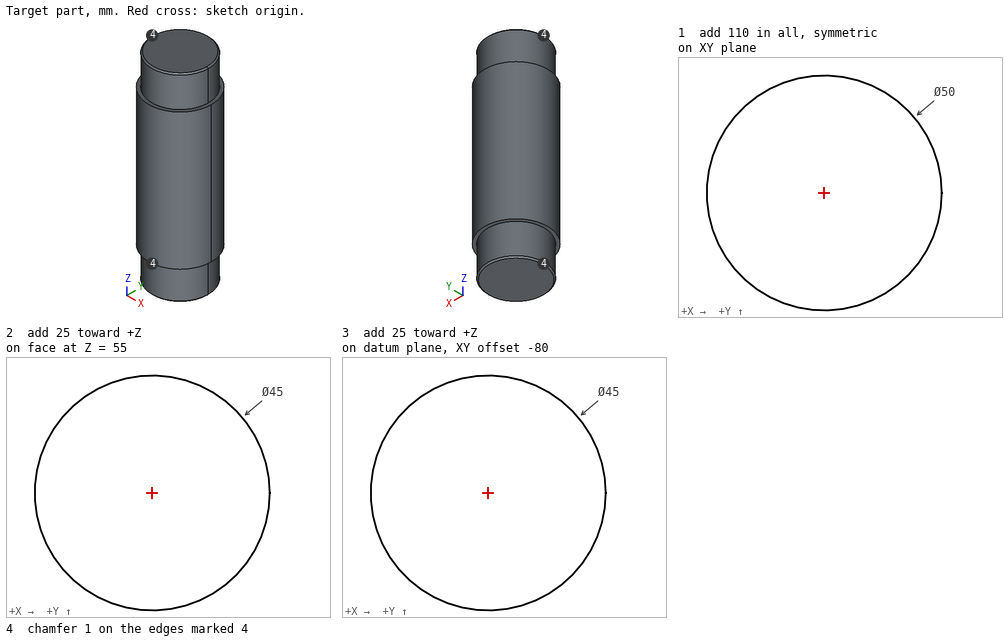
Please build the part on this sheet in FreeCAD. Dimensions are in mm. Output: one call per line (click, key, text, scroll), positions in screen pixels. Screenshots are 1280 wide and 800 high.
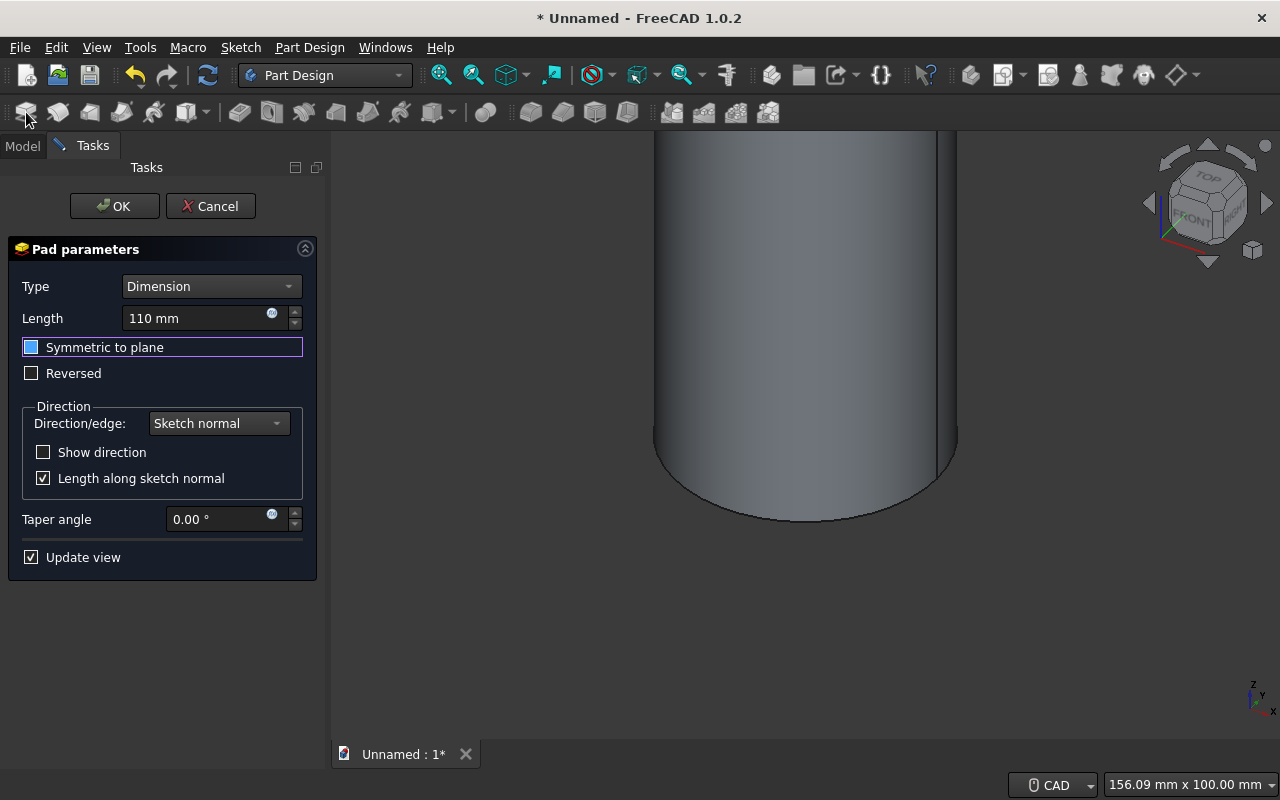
click(30, 347)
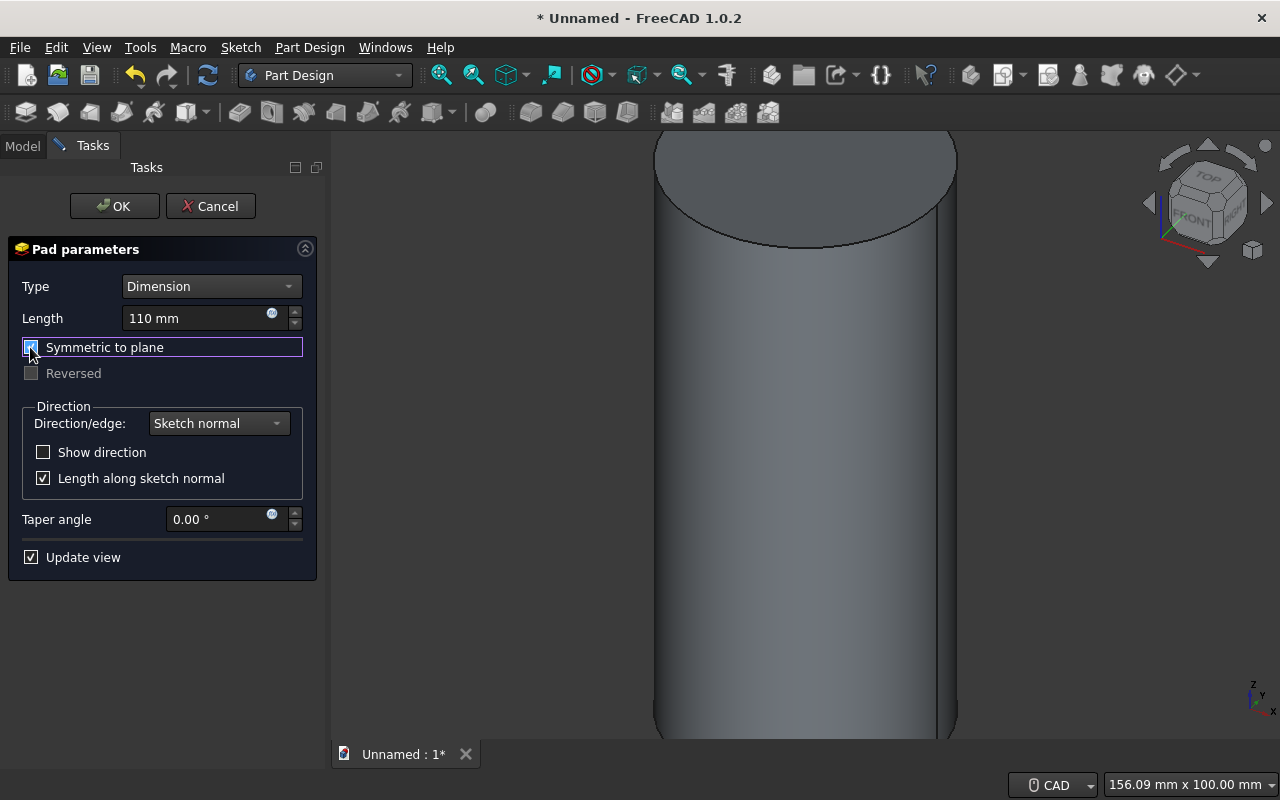
click(115, 206)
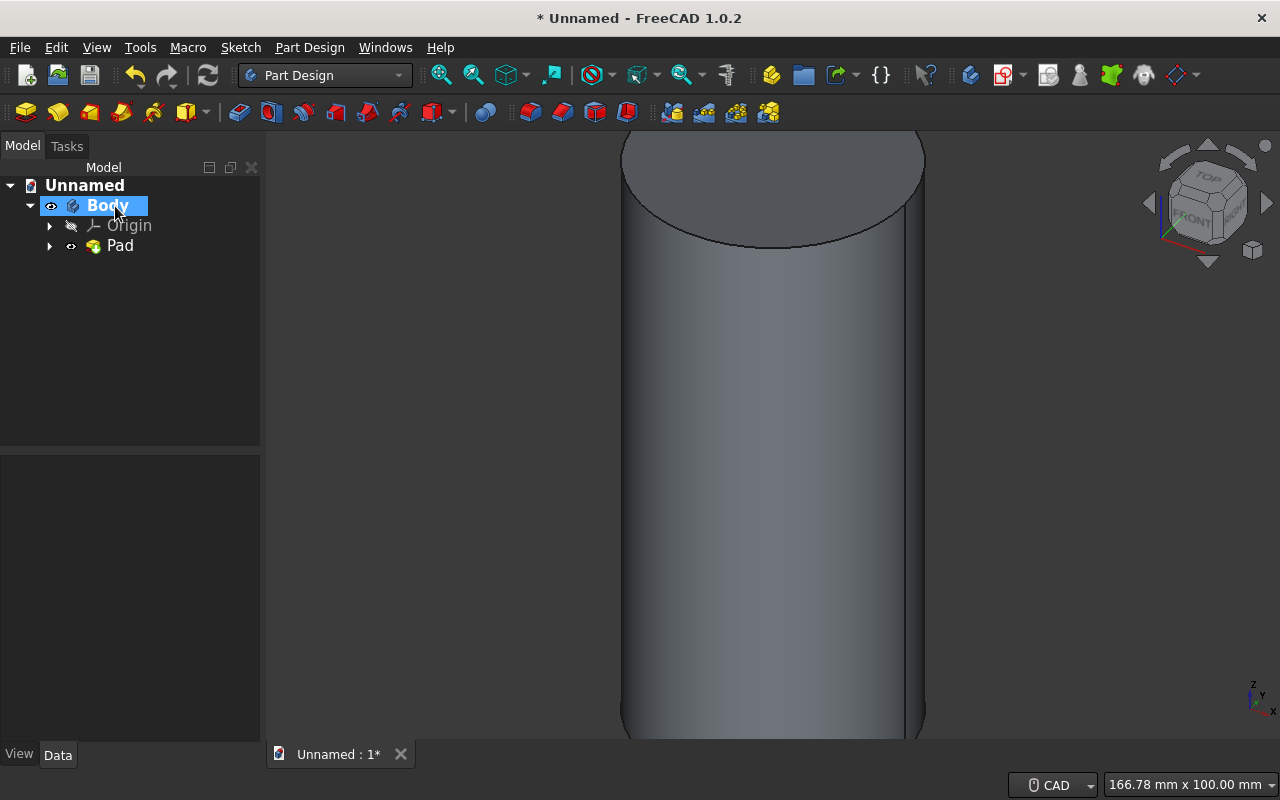
click(442, 76)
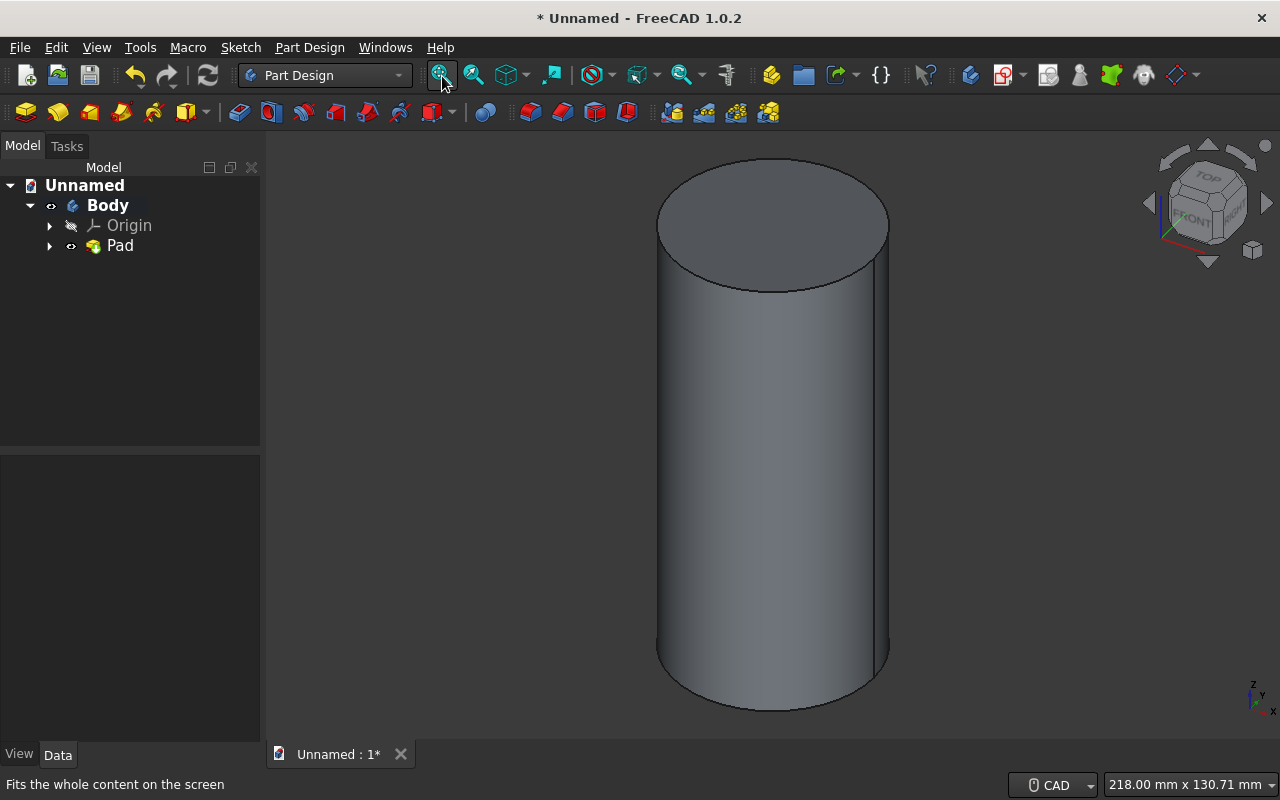
click(773, 224)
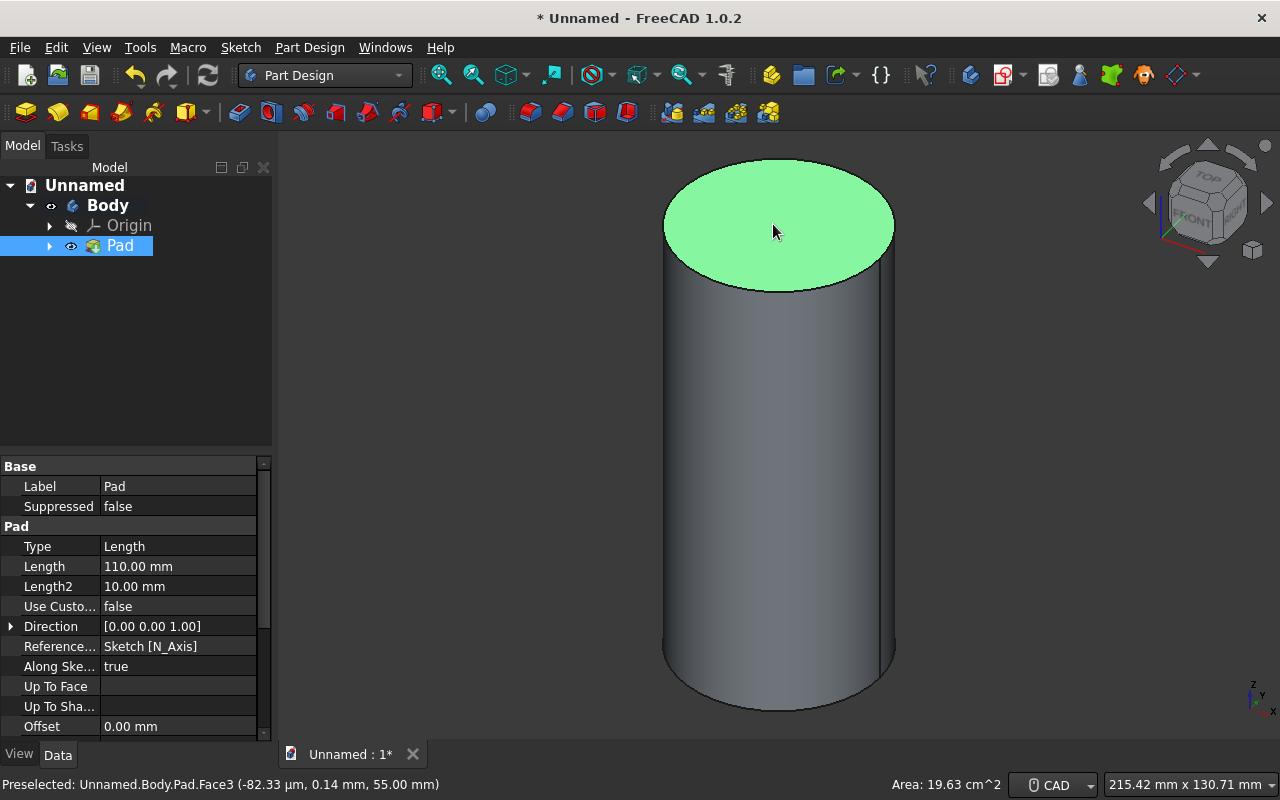
click(1004, 76)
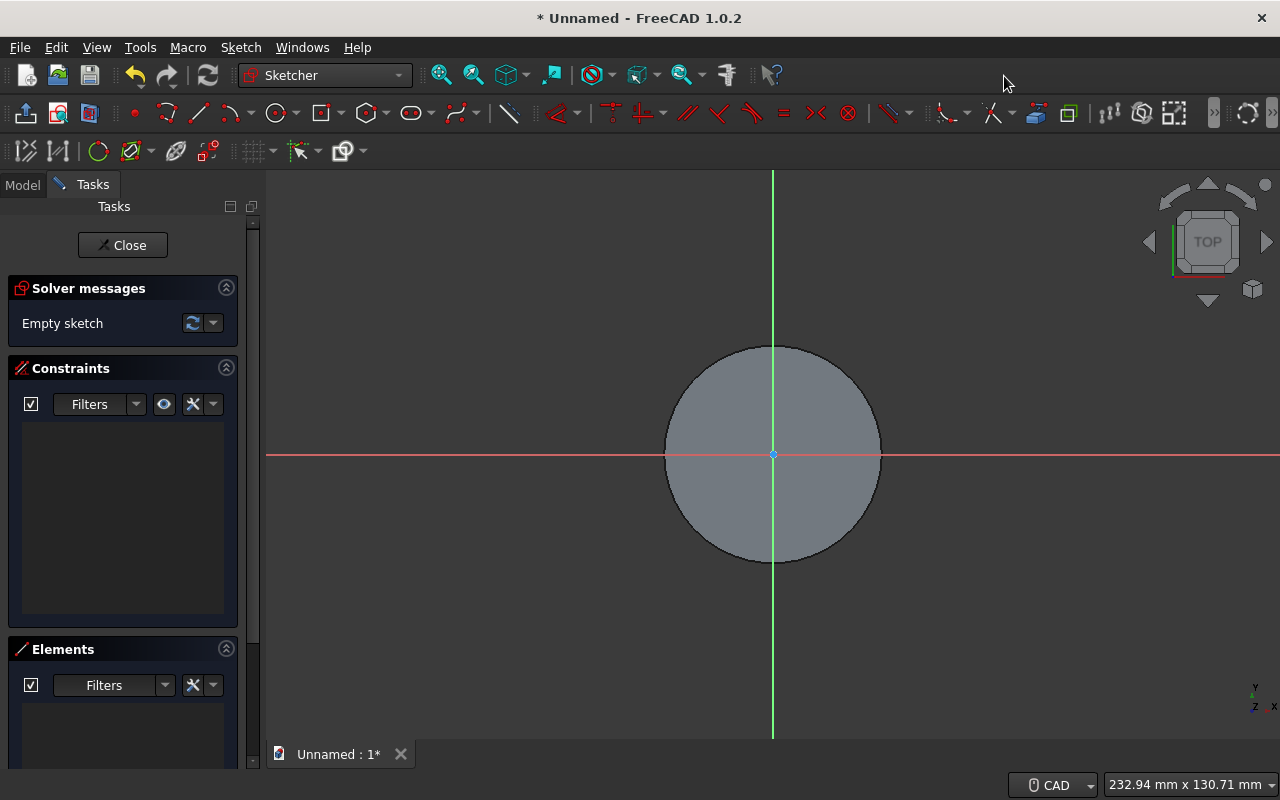
scroll(856, 454, up, 3)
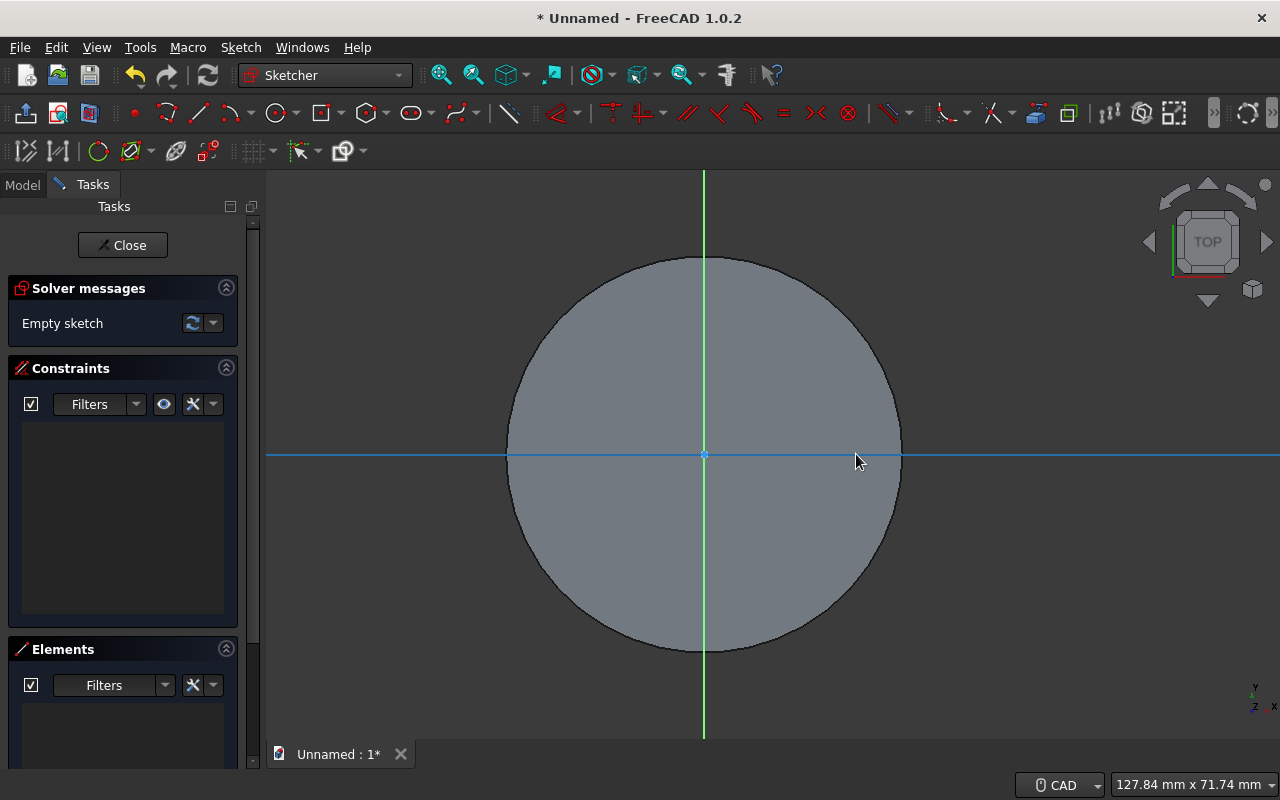
key(g)
key(c)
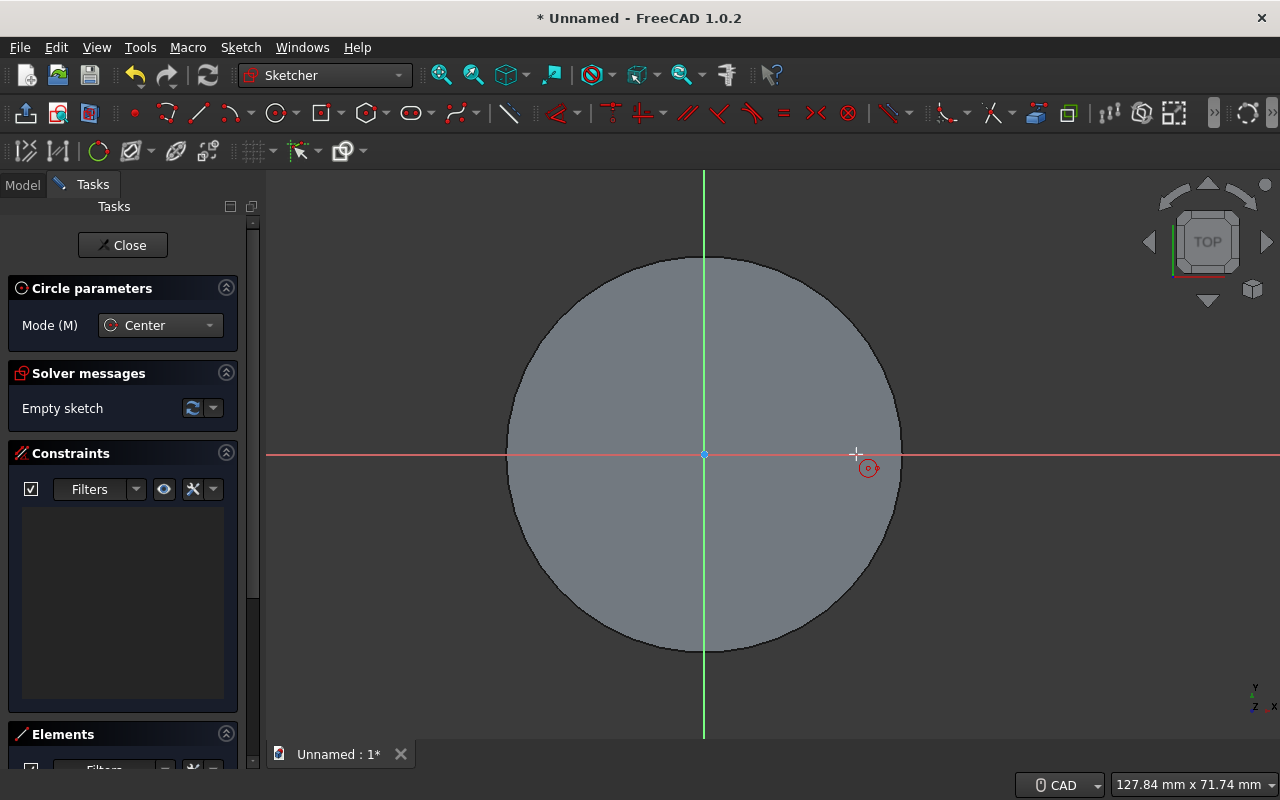
click(704, 454)
move(830, 328)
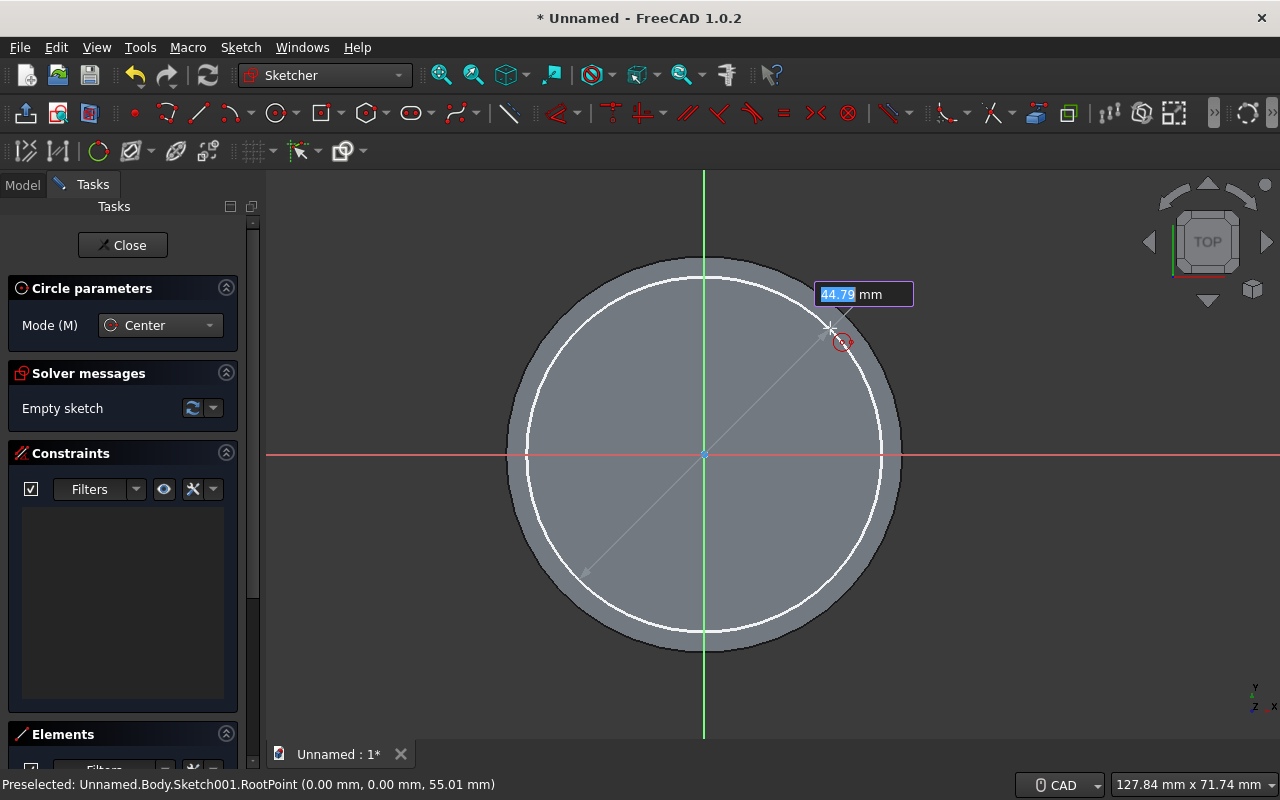
text(45)
key(Return)
key(Escape)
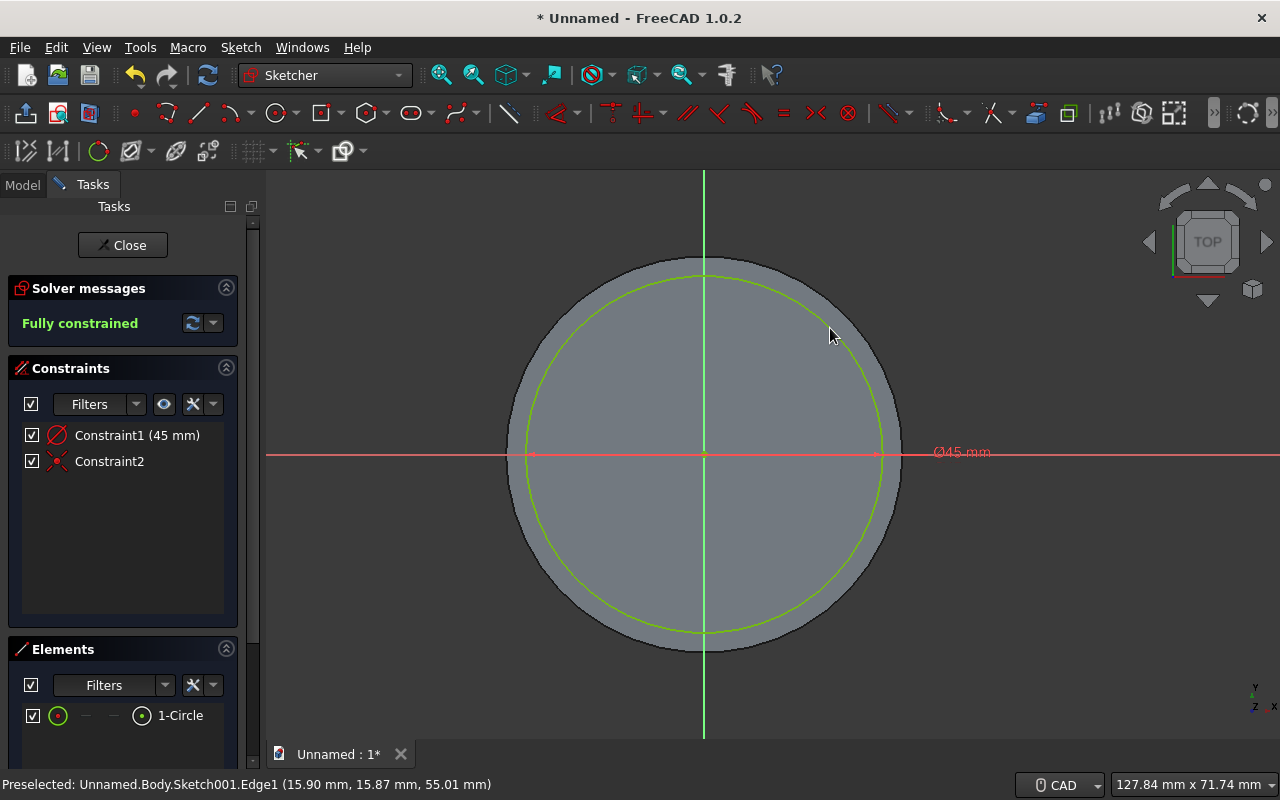
click(123, 245)